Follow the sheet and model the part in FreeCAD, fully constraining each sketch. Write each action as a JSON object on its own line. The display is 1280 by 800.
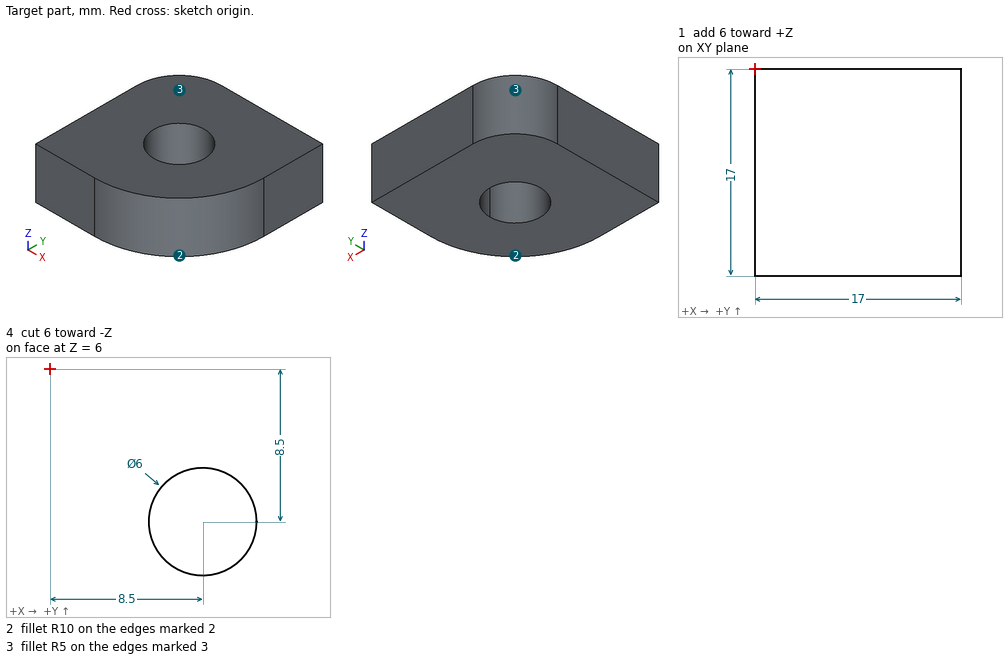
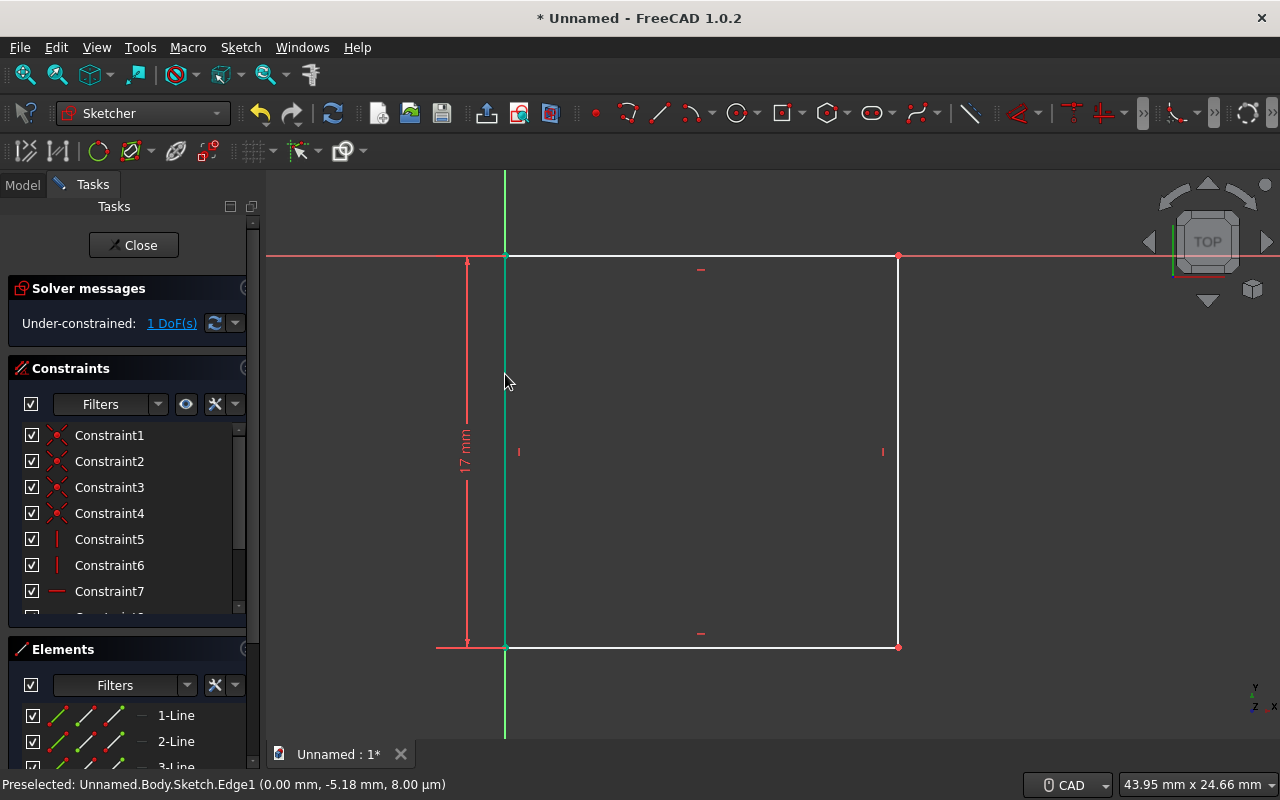
{"action": "left_click", "coordinate": [623, 648]}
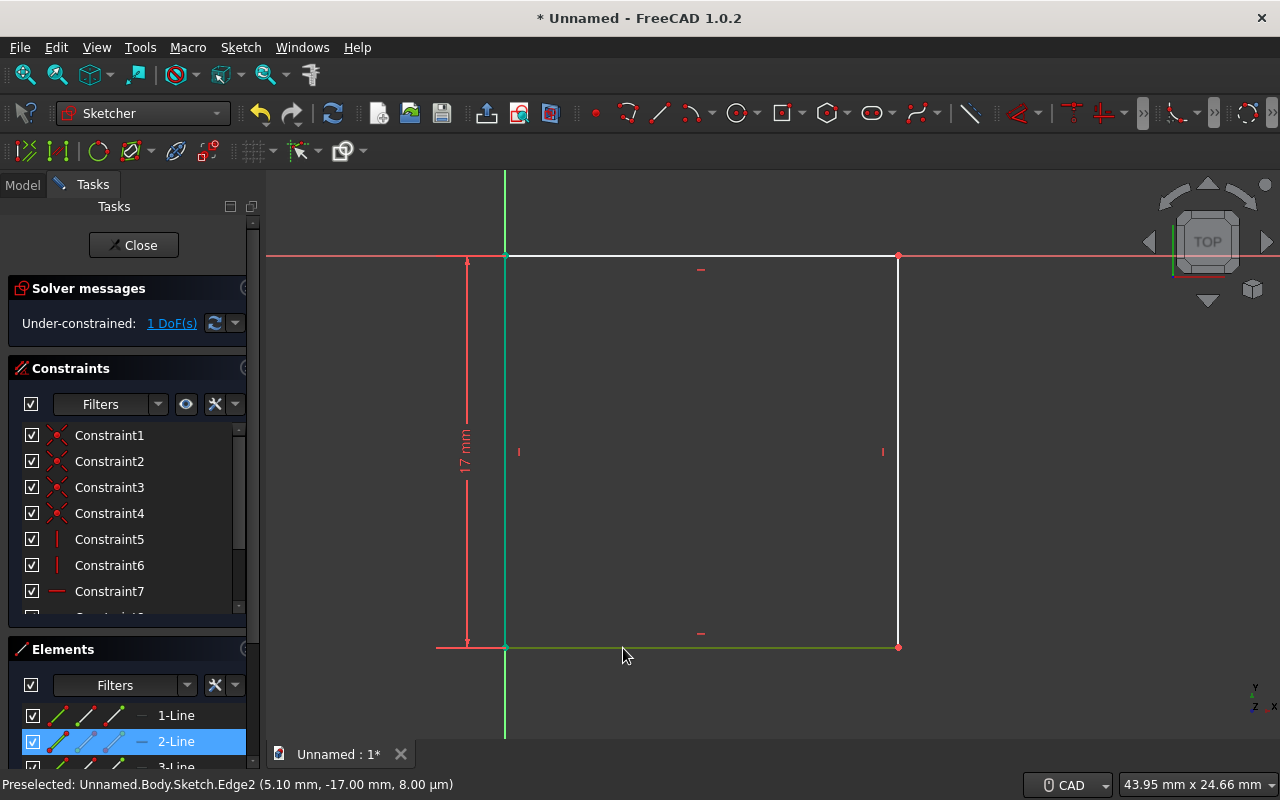
{"action": "key", "text": "l"}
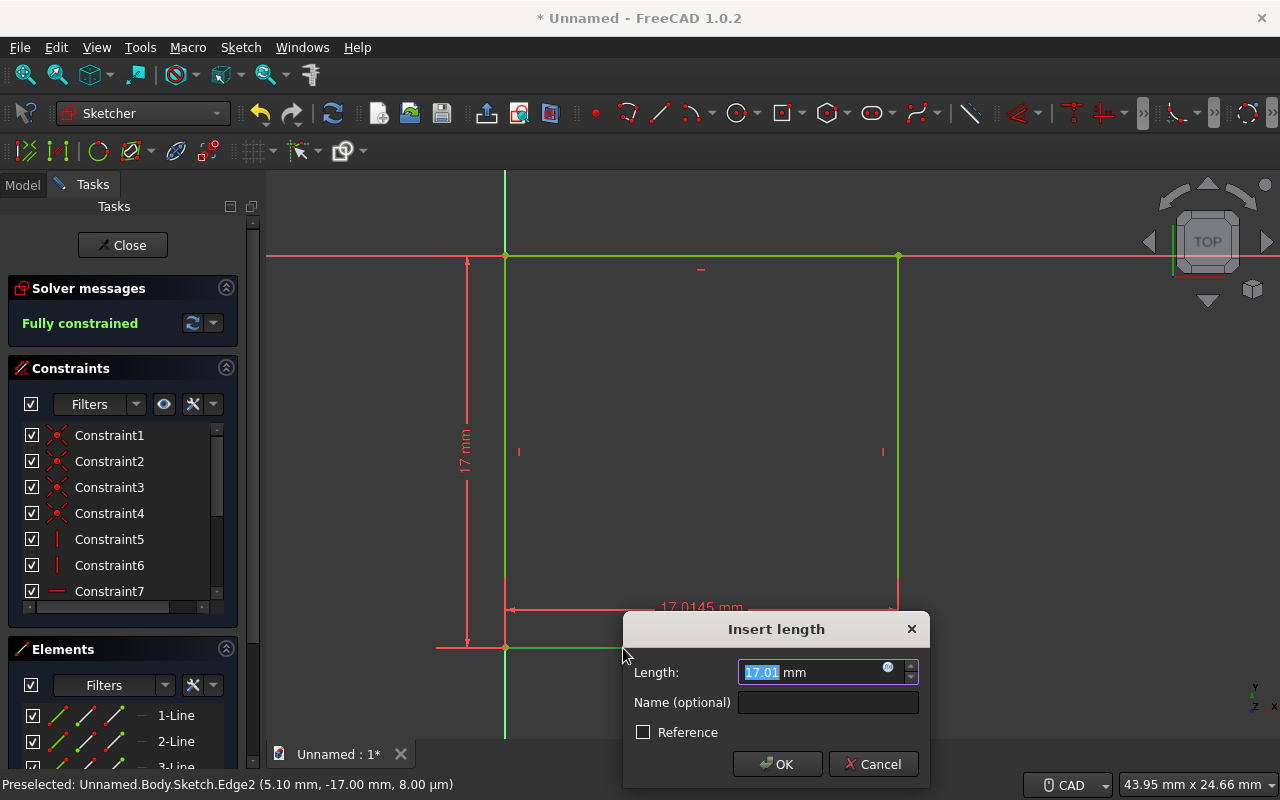
{"action": "type", "text": "17"}
{"action": "key", "text": "Return"}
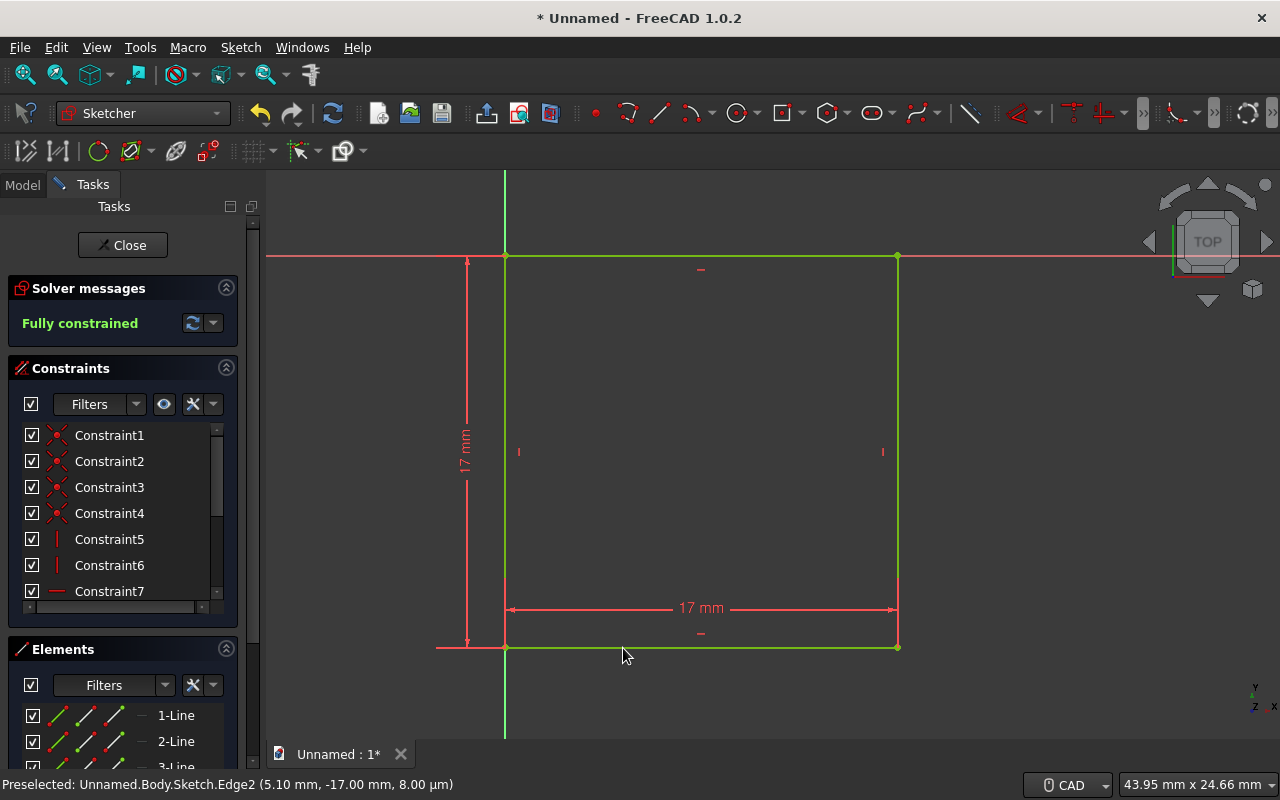
{"action": "left_click", "coordinate": [123, 245]}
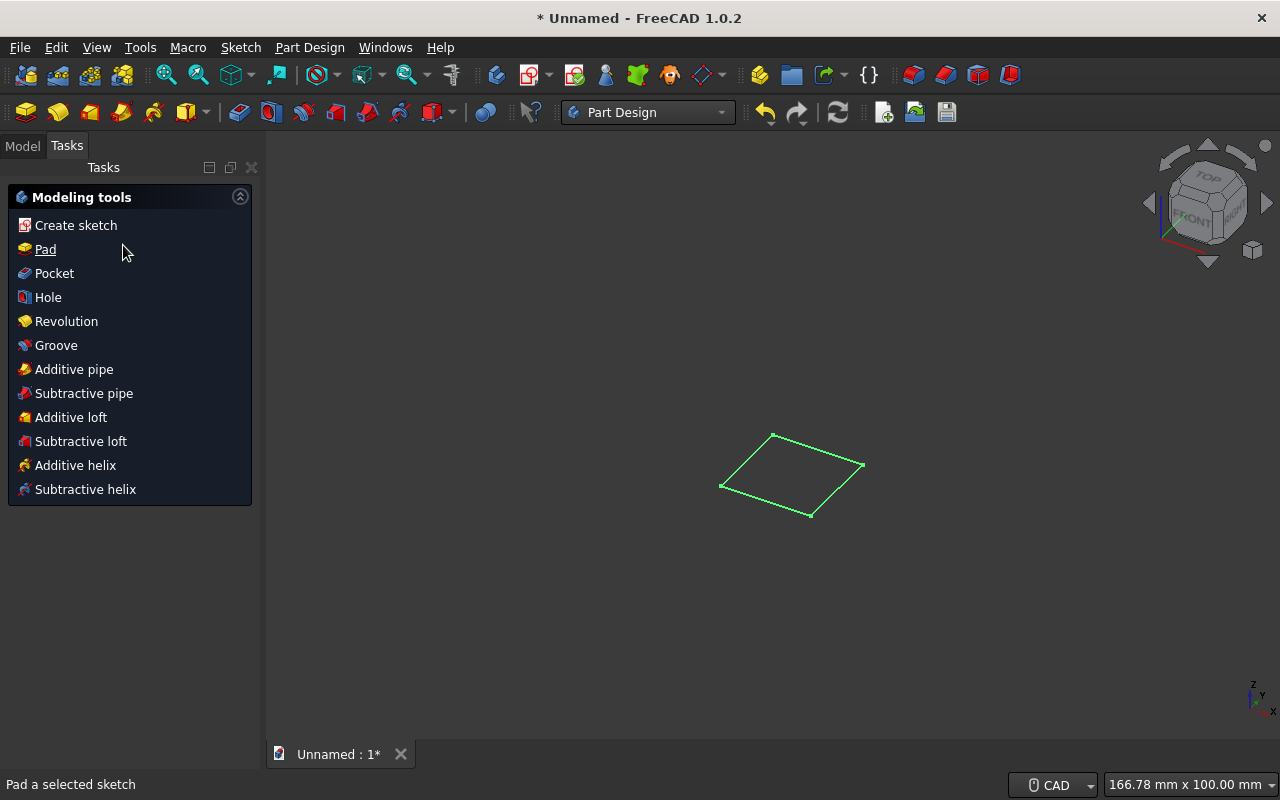
{"action": "left_click", "coordinate": [26, 112]}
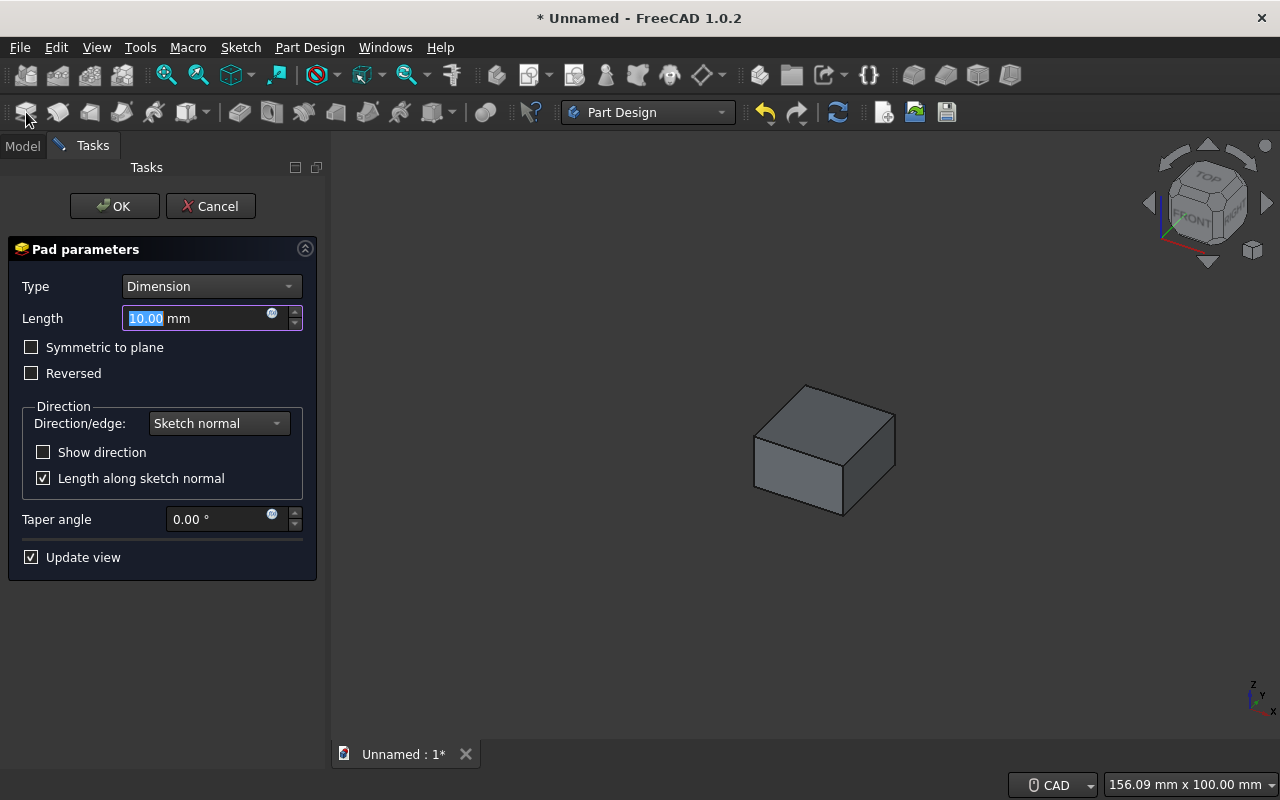
{"action": "type", "text": "6"}
{"action": "key", "text": "Tab"}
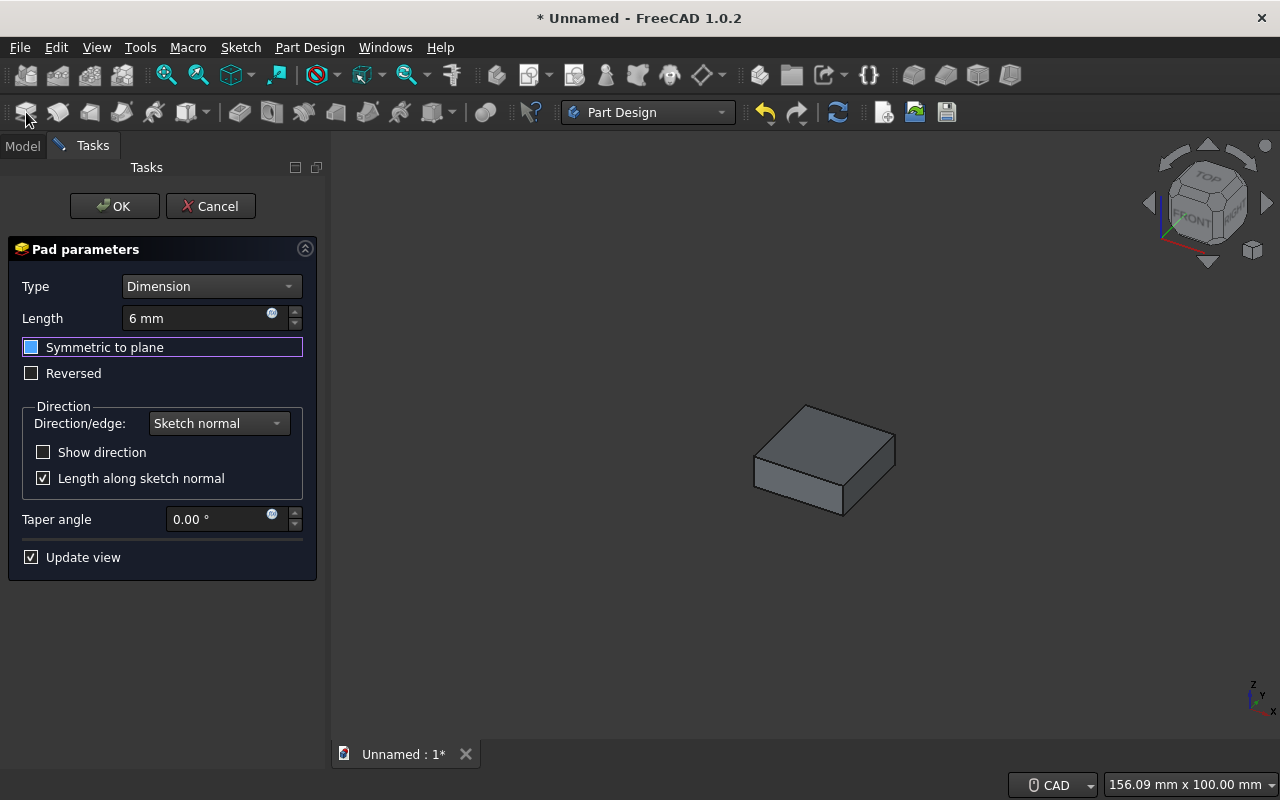
{"action": "left_click", "coordinate": [115, 206]}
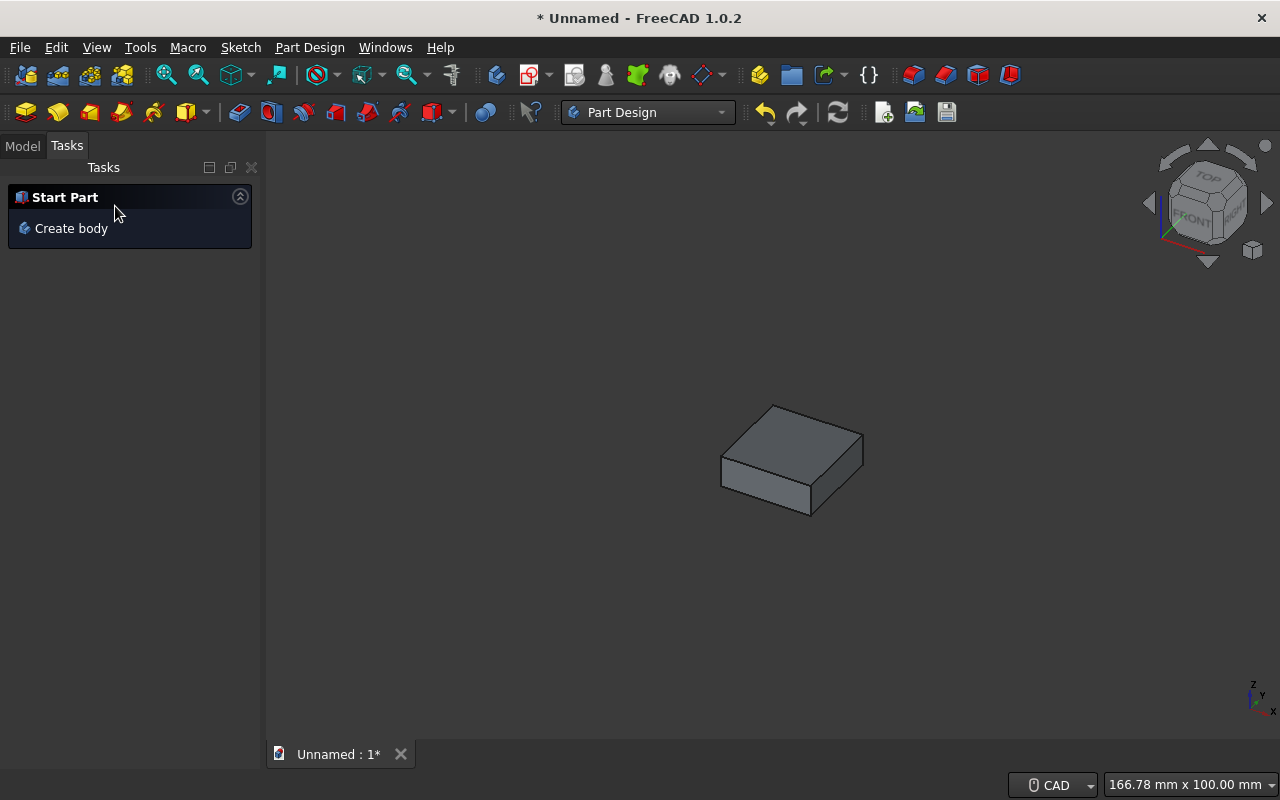
{"action": "left_click", "coordinate": [168, 76]}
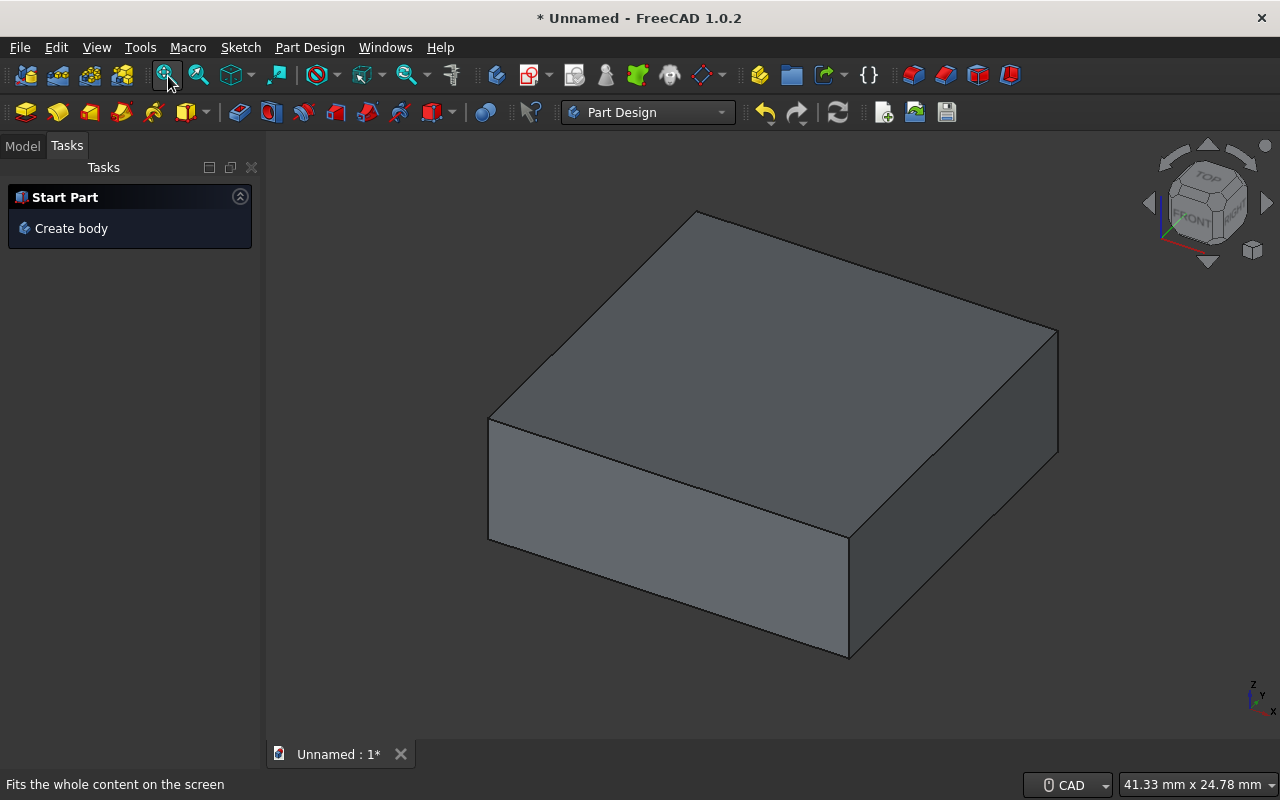
{"action": "left_click", "coordinate": [849, 597]}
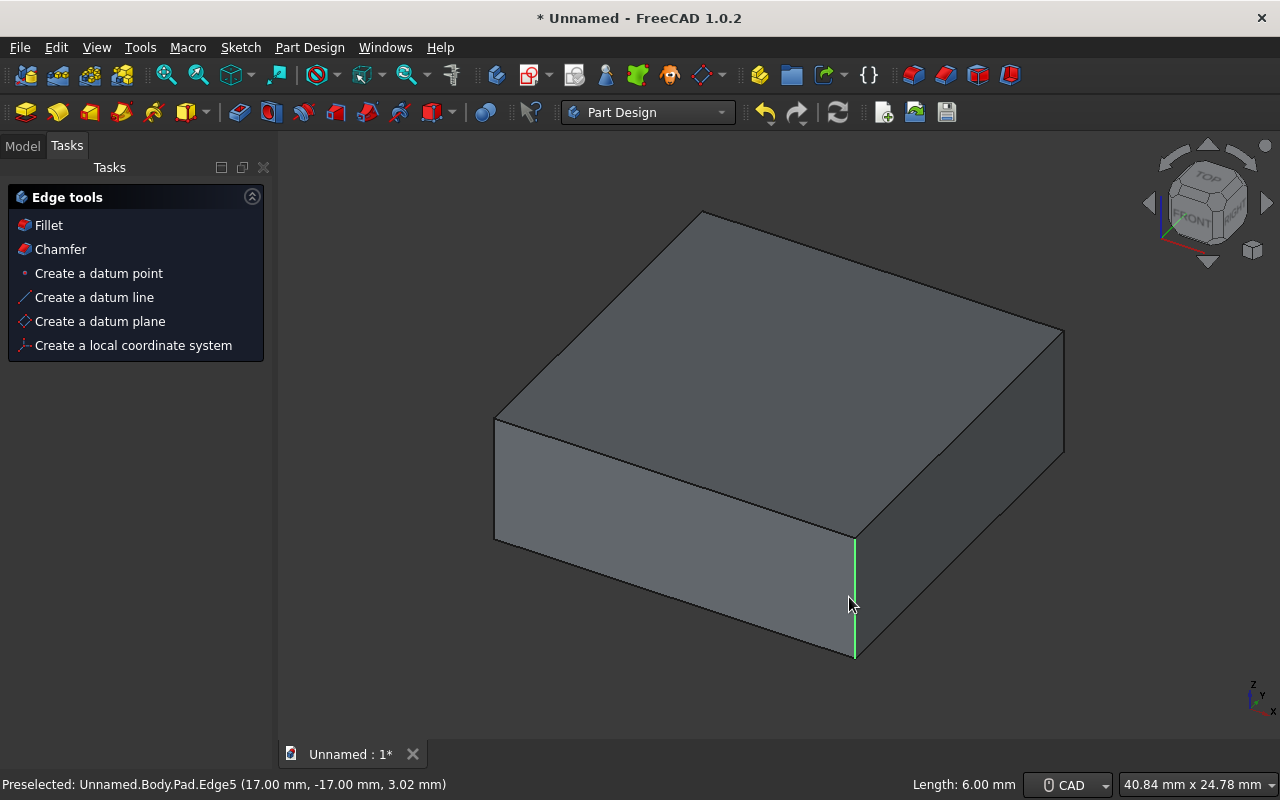
{"action": "left_click", "coordinate": [914, 76]}